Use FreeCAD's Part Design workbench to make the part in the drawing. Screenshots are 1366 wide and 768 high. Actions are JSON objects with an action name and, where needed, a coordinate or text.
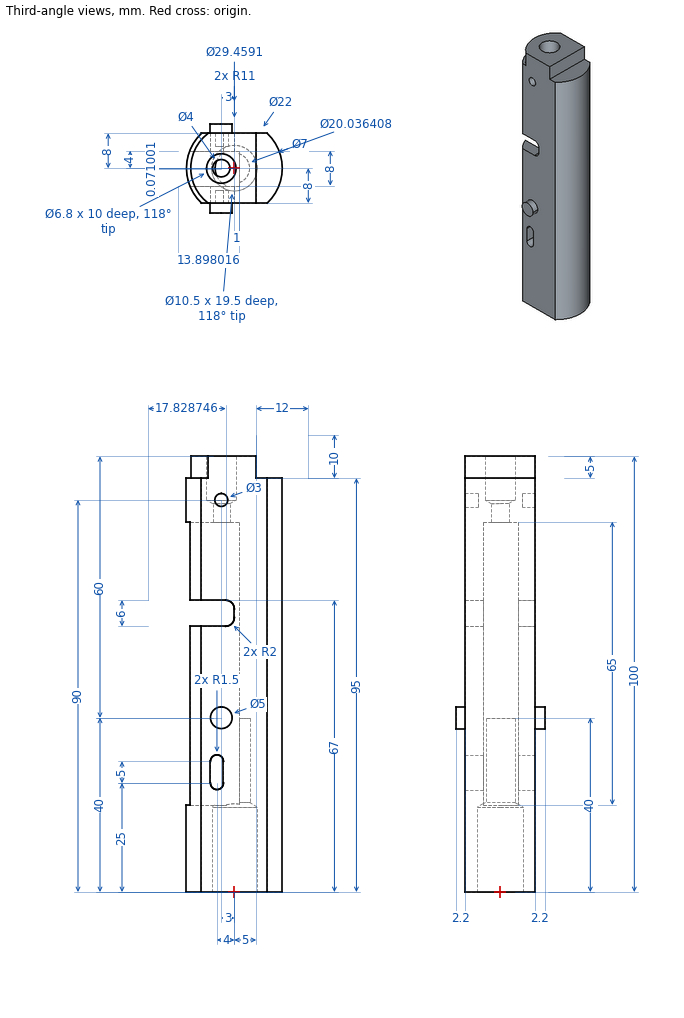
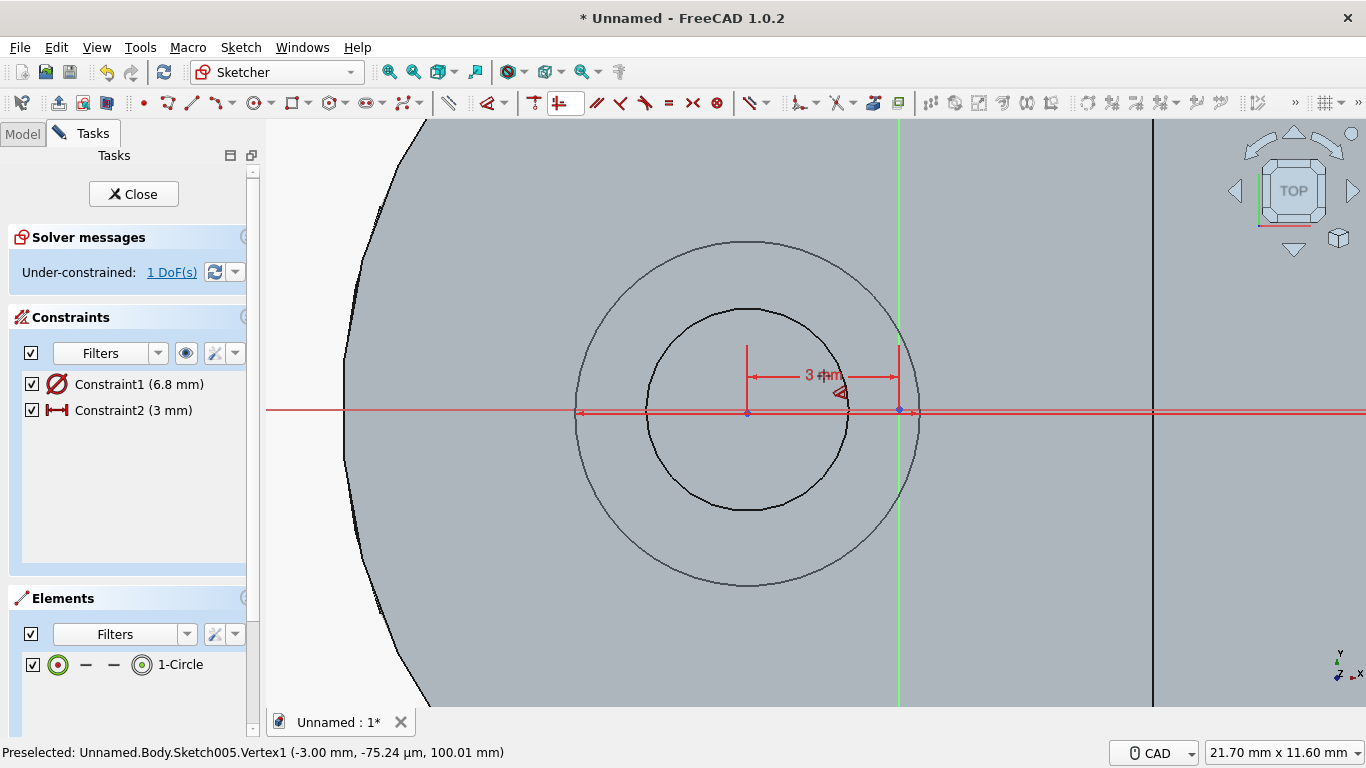
{"action": "scroll", "coordinate": [747, 414], "scroll_direction": "up", "scroll_amount": 13}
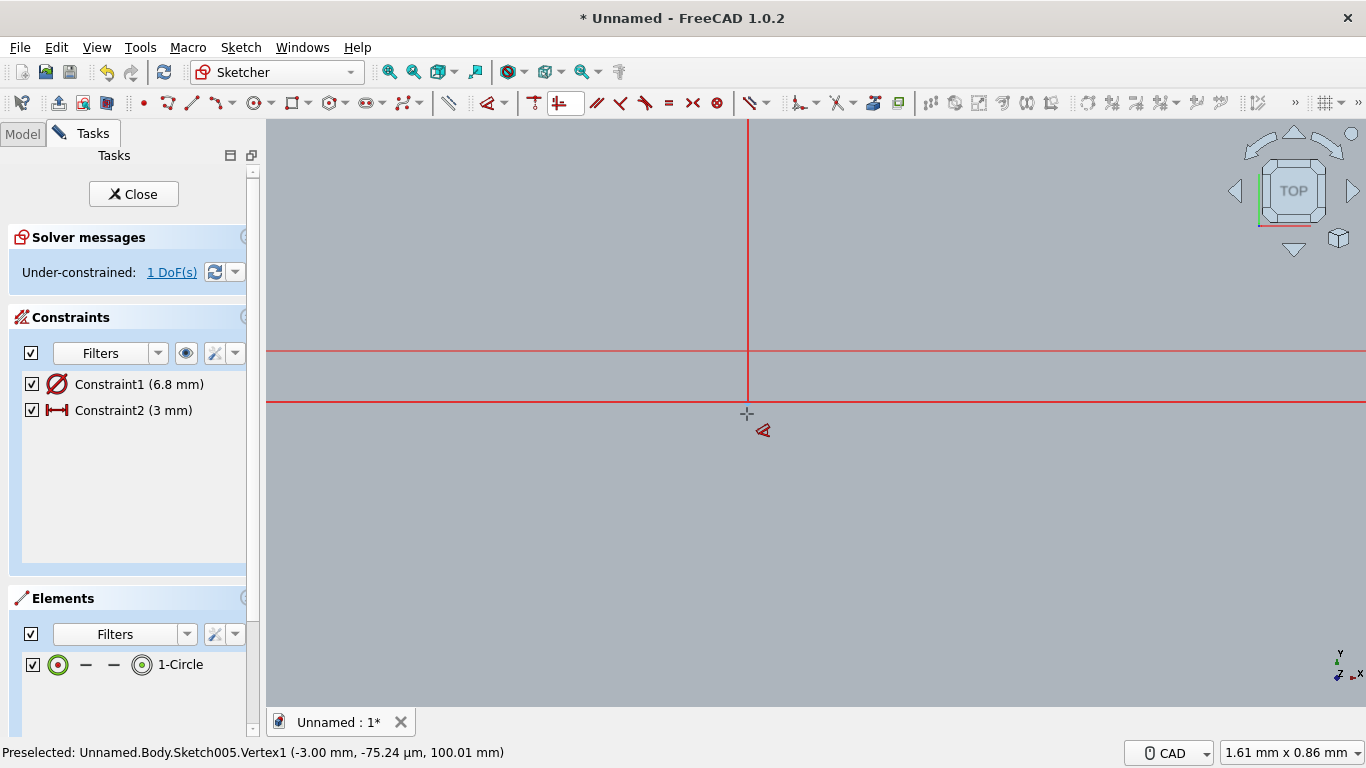
{"action": "left_click", "coordinate": [748, 402]}
{"action": "left_click", "coordinate": [714, 377]}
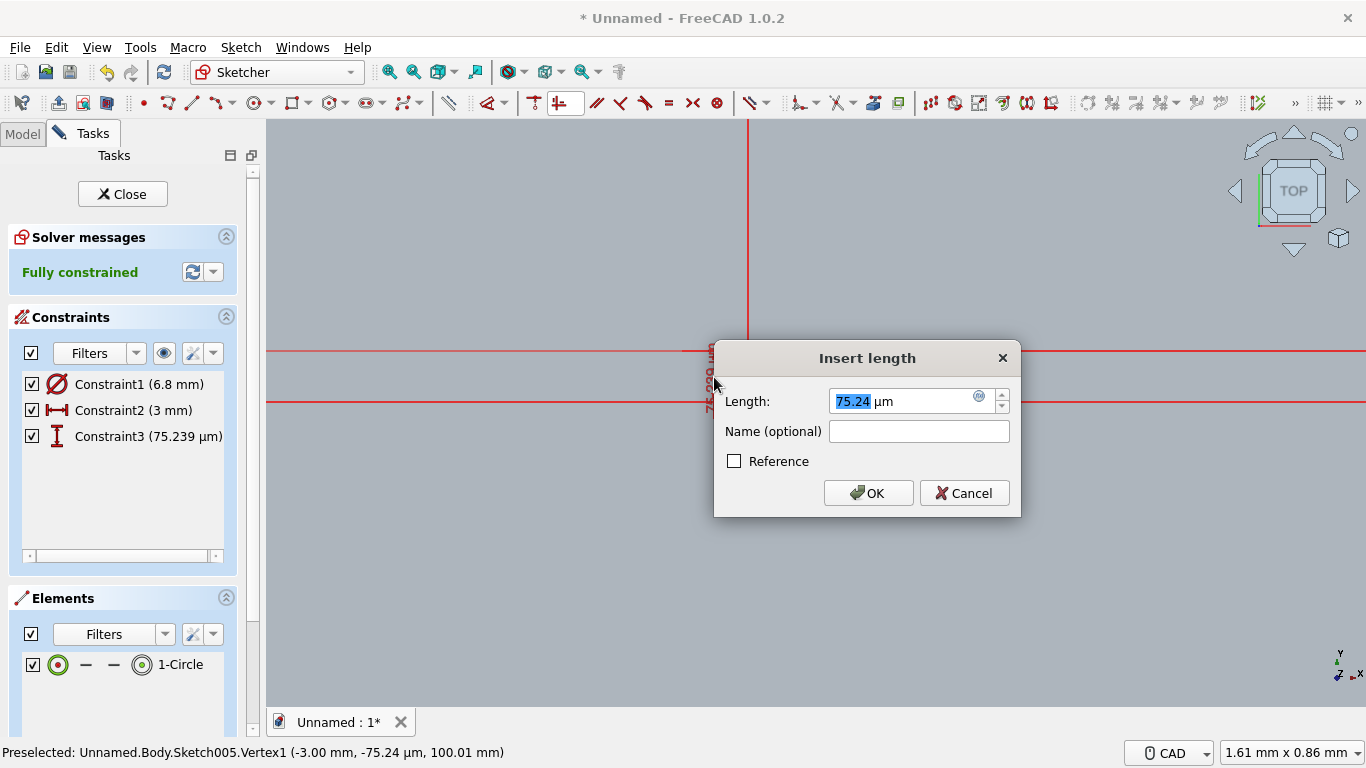
{"action": "key", "text": "ctrl+a"}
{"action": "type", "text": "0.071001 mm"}
{"action": "key", "text": "Return"}
{"action": "key", "text": "Escape"}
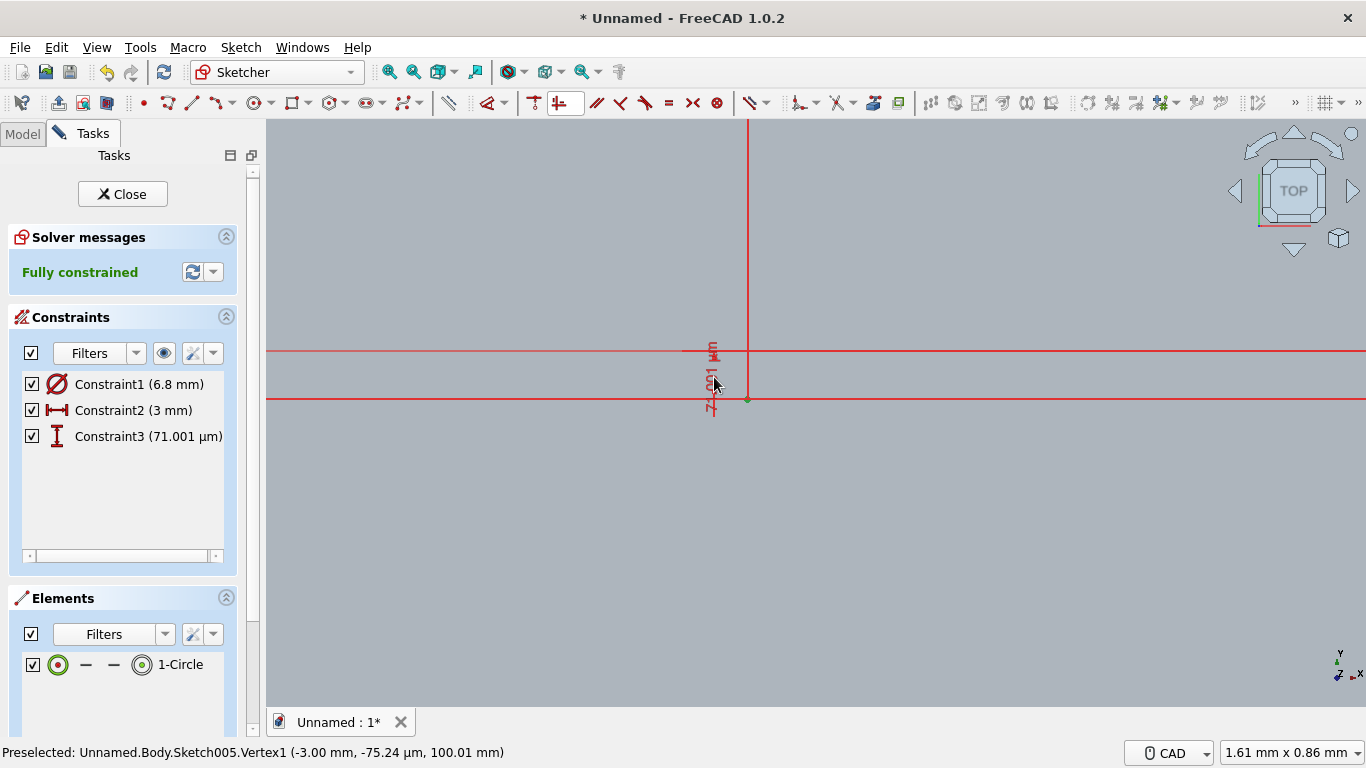
{"action": "left_click", "coordinate": [123, 194]}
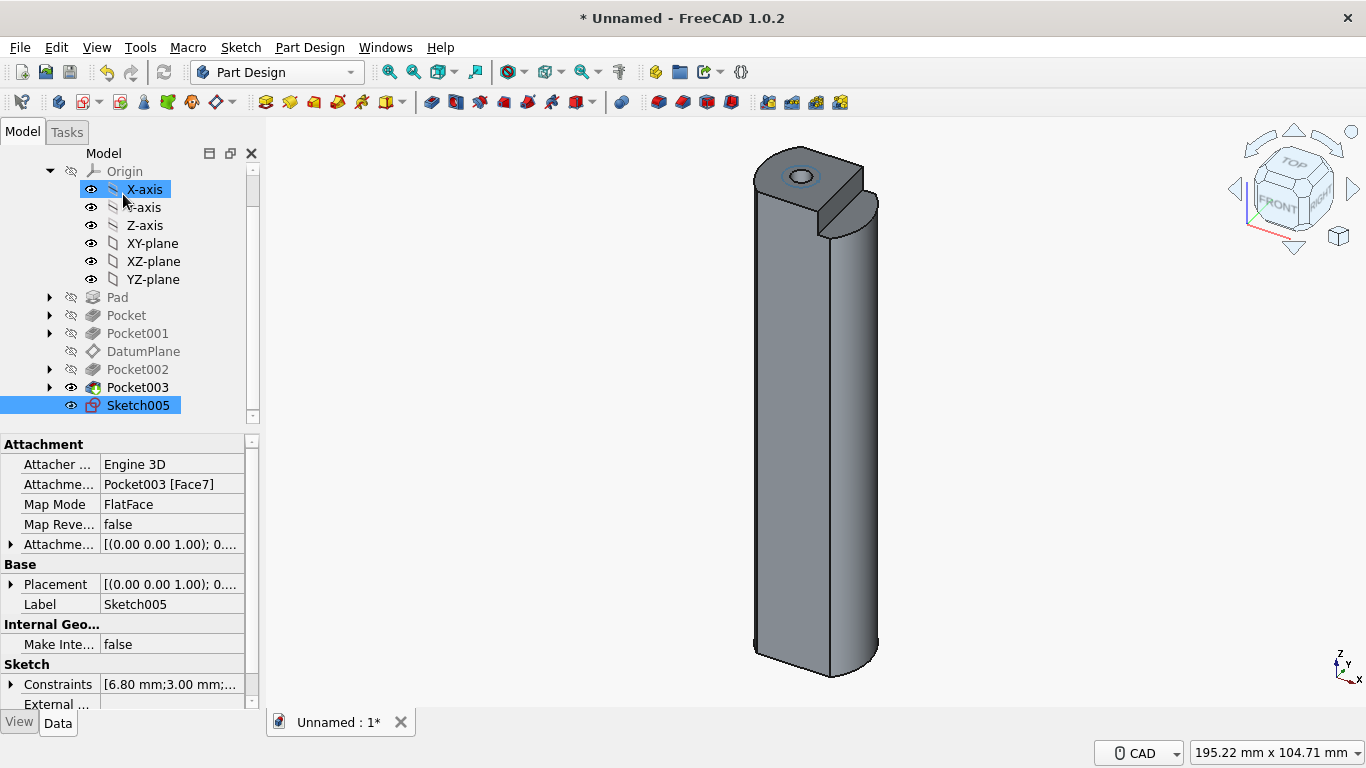
{"action": "left_click", "coordinate": [456, 102]}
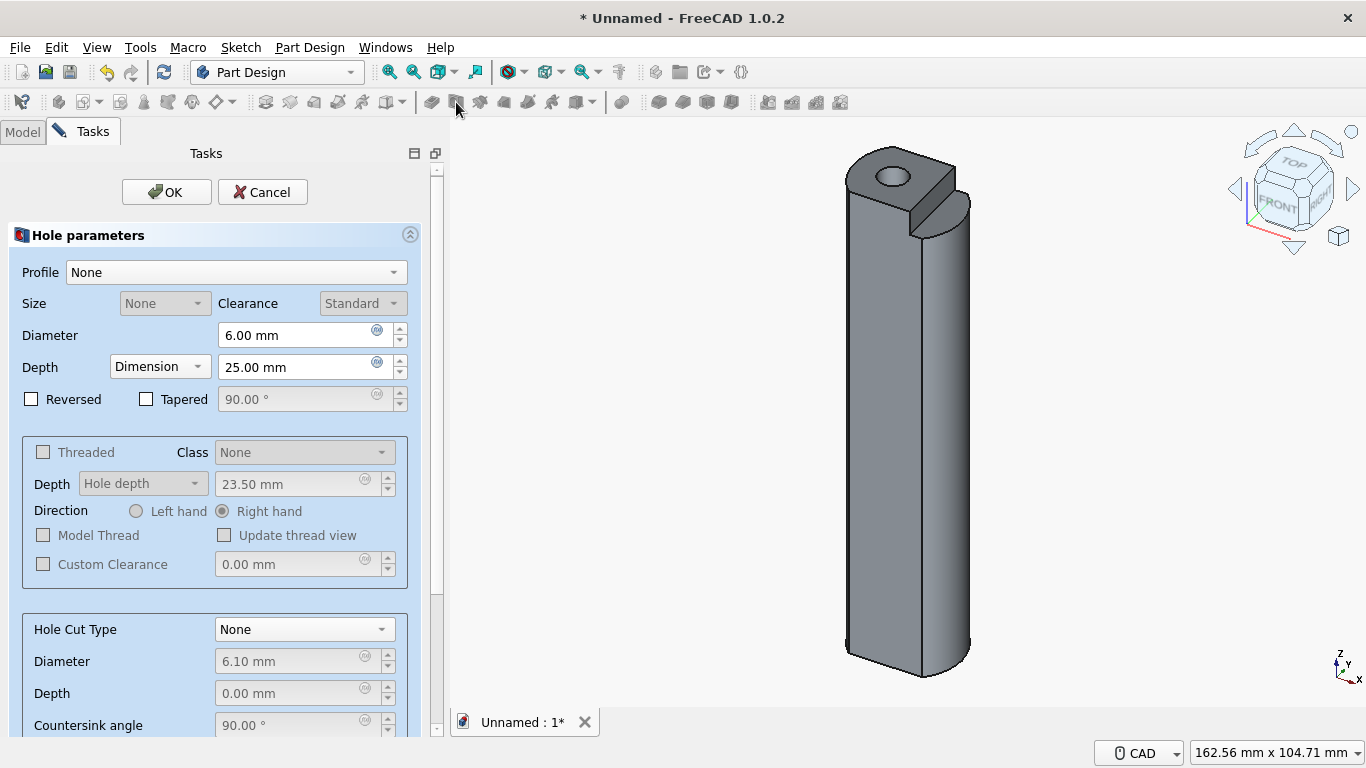
{"action": "triple_click", "coordinate": [305, 335]}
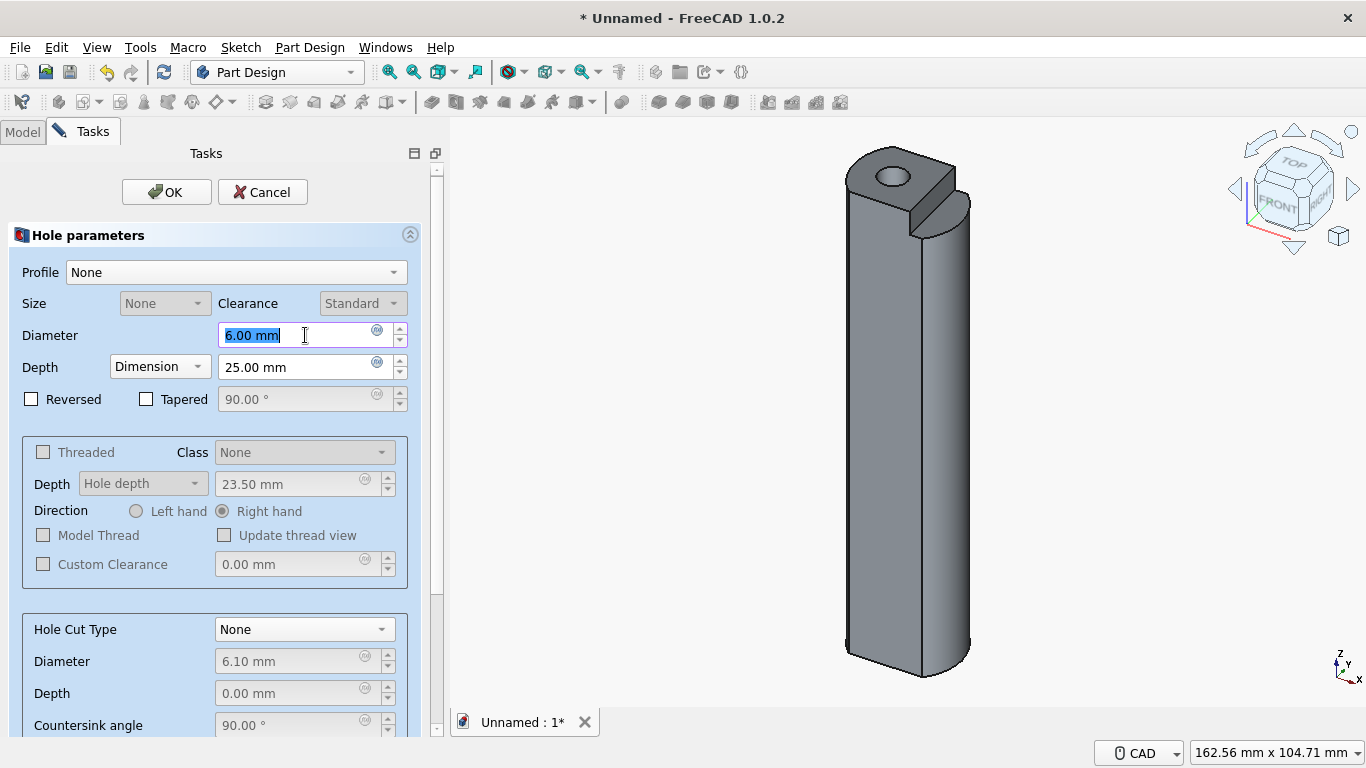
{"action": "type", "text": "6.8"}
{"action": "key", "text": "Tab"}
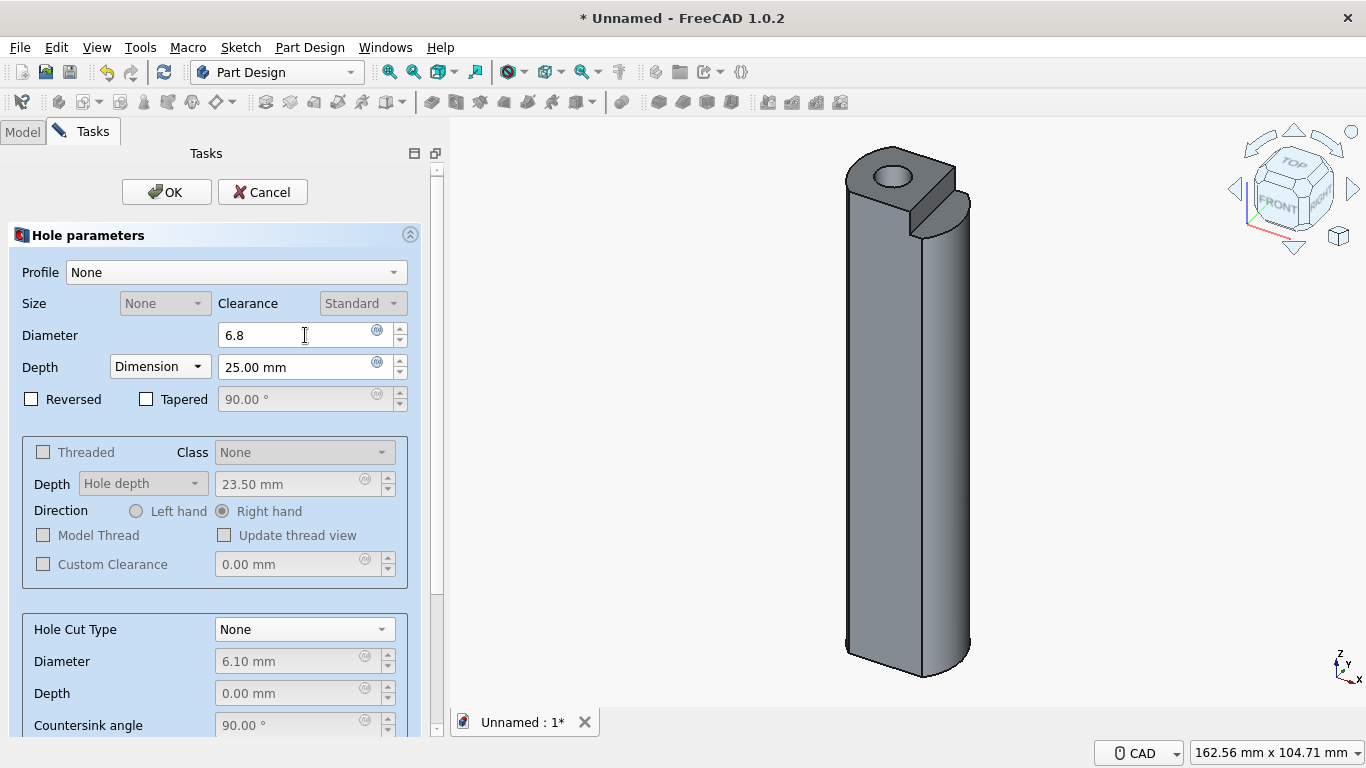
{"action": "triple_click", "coordinate": [305, 367]}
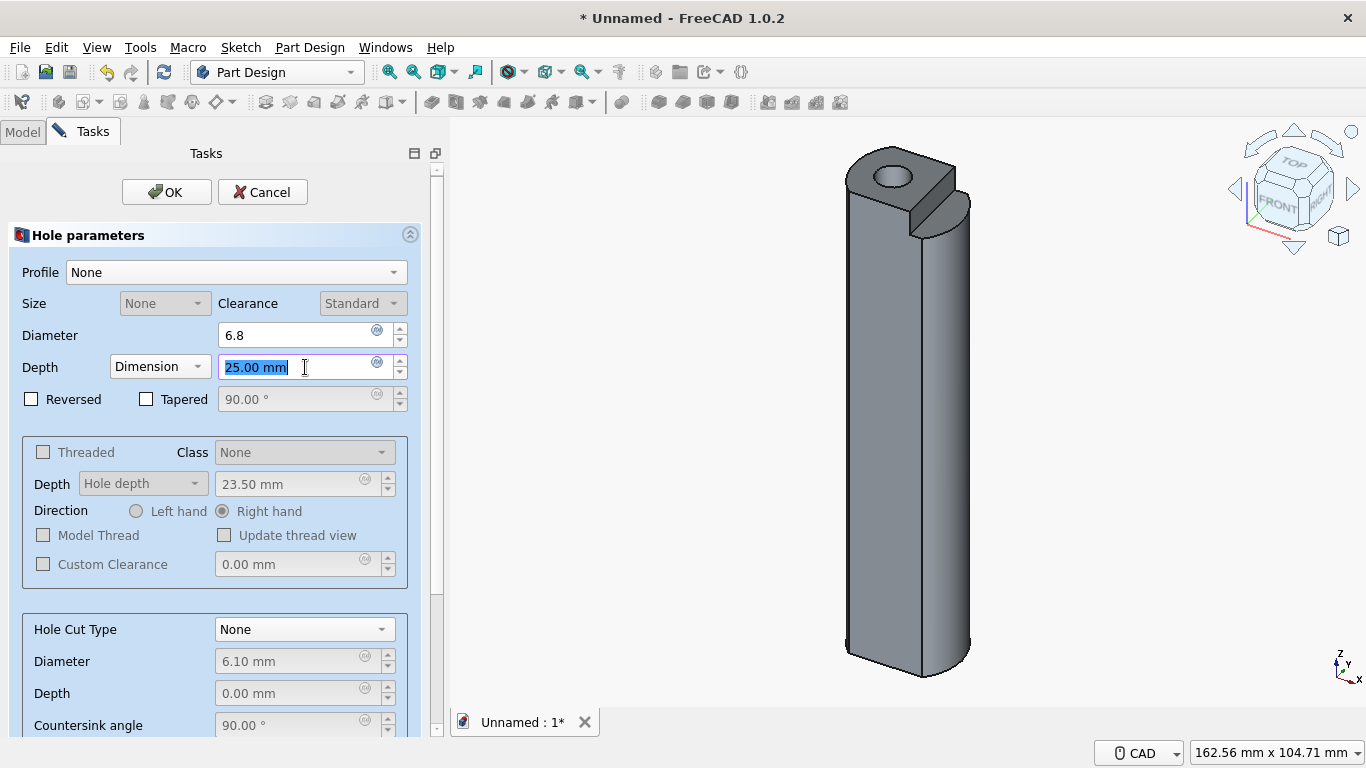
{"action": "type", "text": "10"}
{"action": "key", "text": "Tab"}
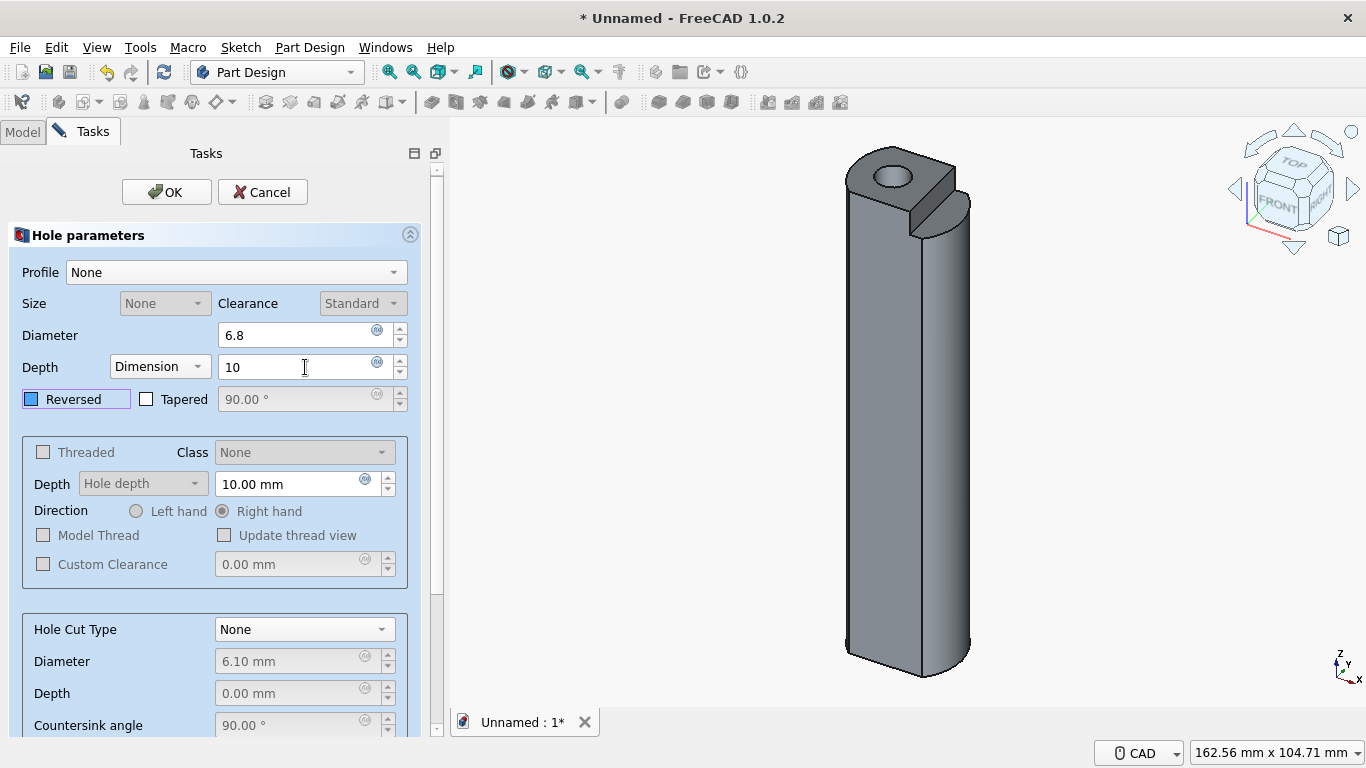
{"action": "left_click", "coordinate": [167, 192]}